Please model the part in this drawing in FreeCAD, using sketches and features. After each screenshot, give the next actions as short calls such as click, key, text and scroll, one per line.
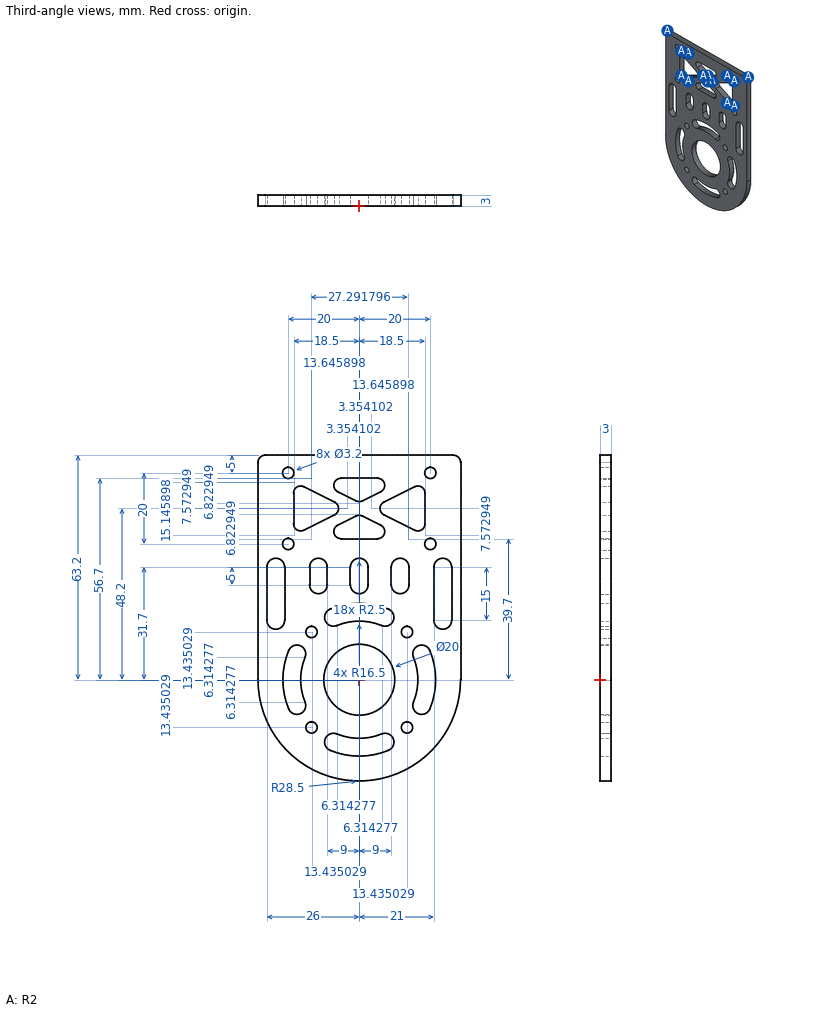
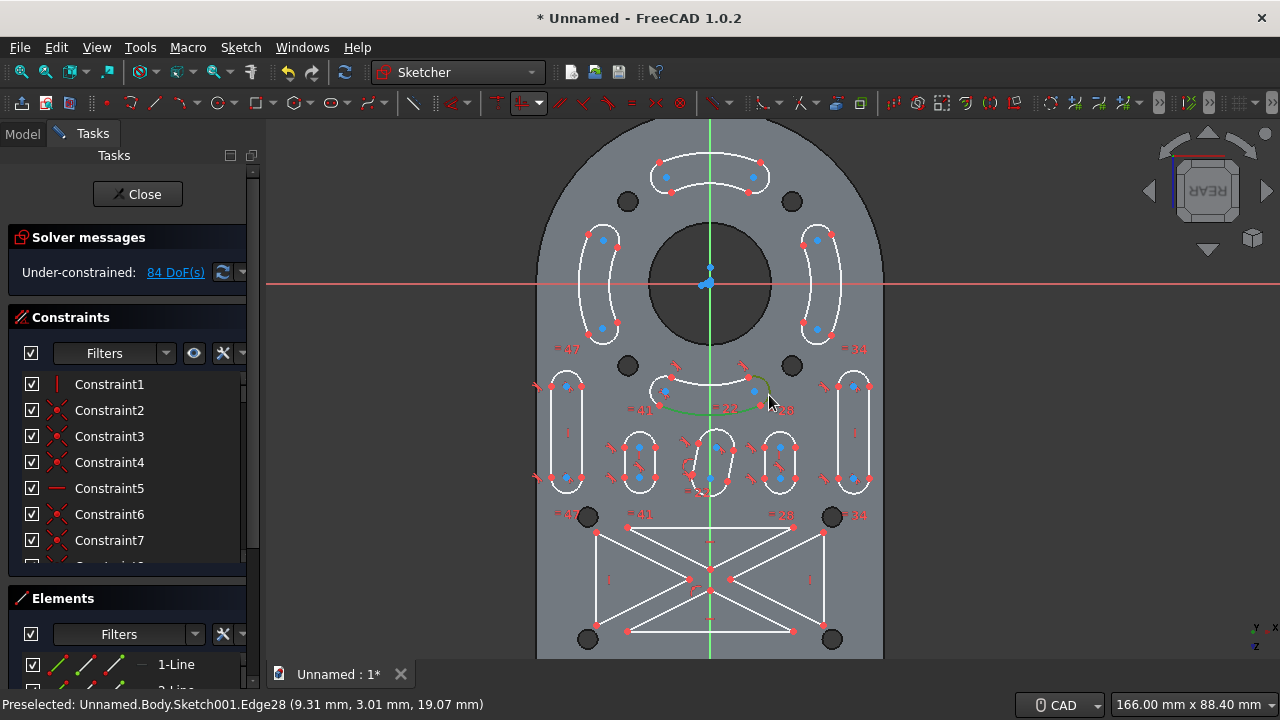
key(t)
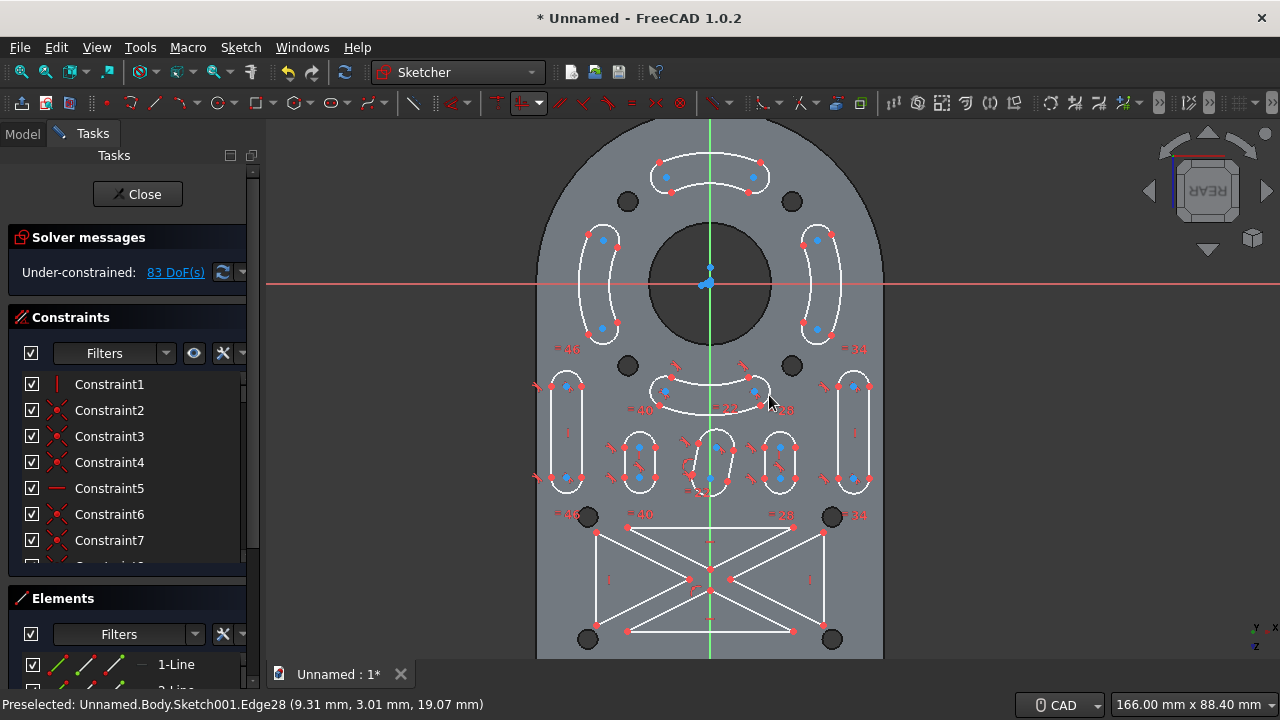
click(611, 269)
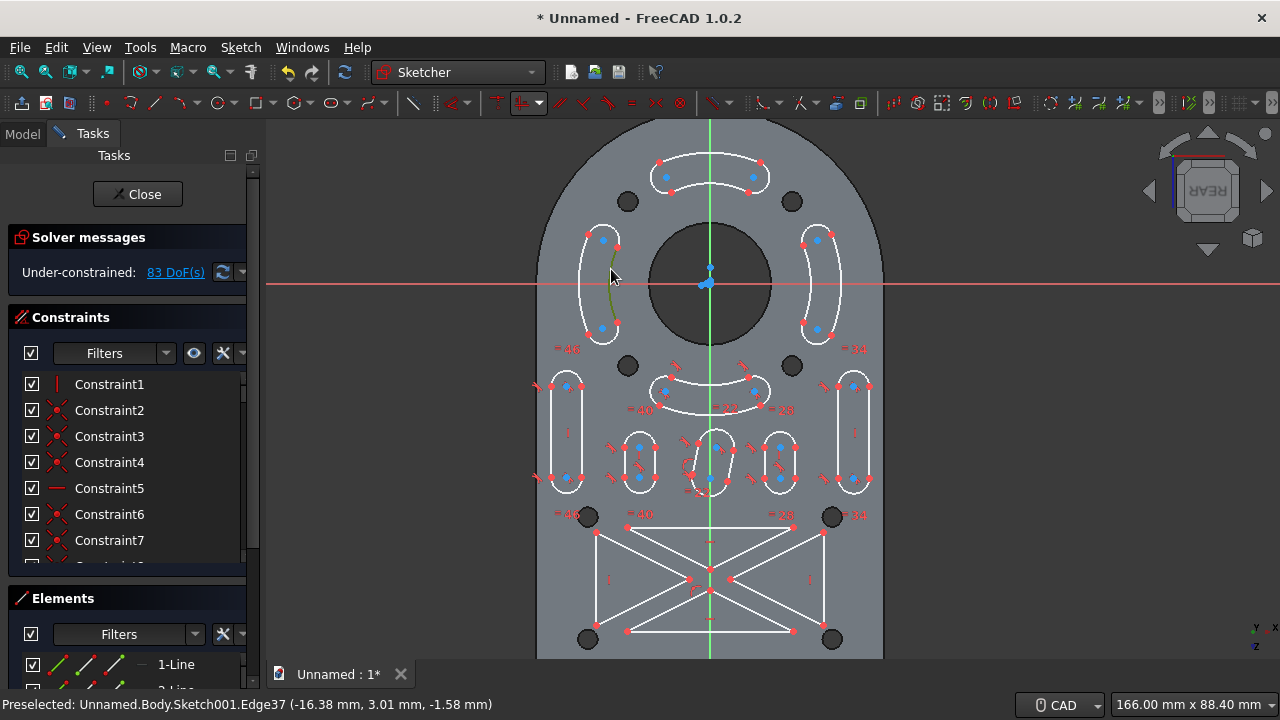
click(617, 233)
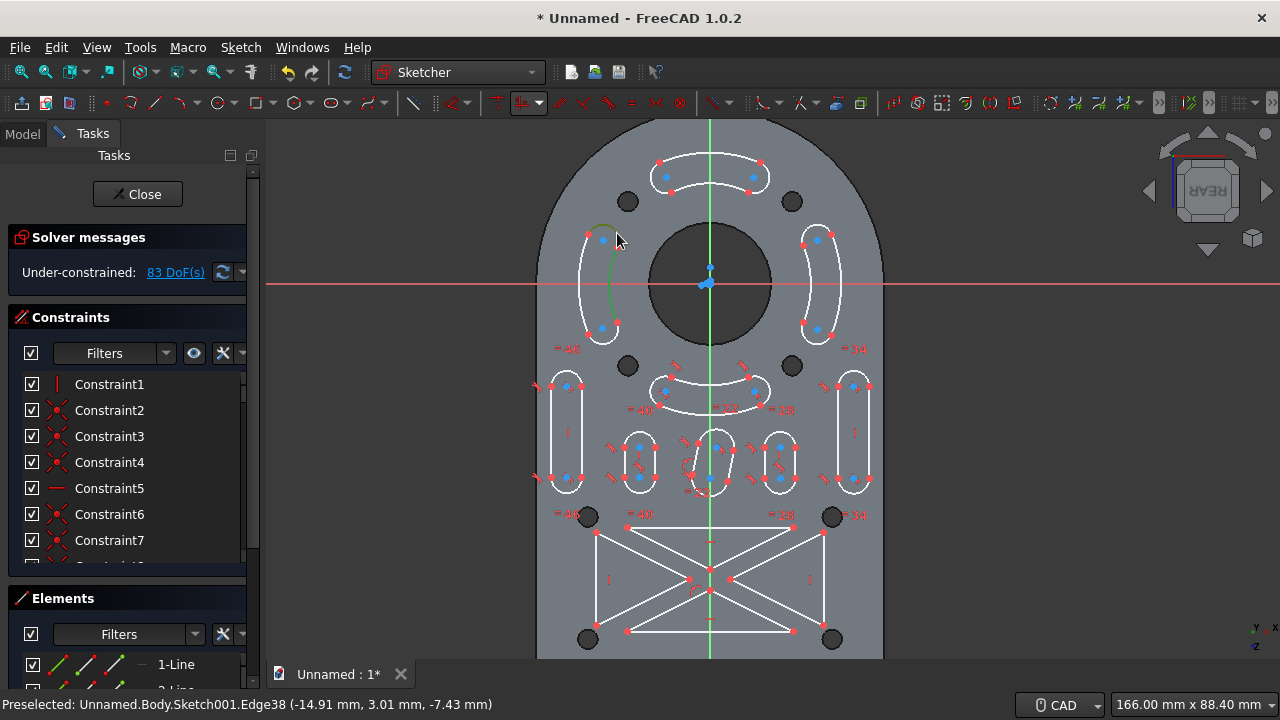
click(608, 104)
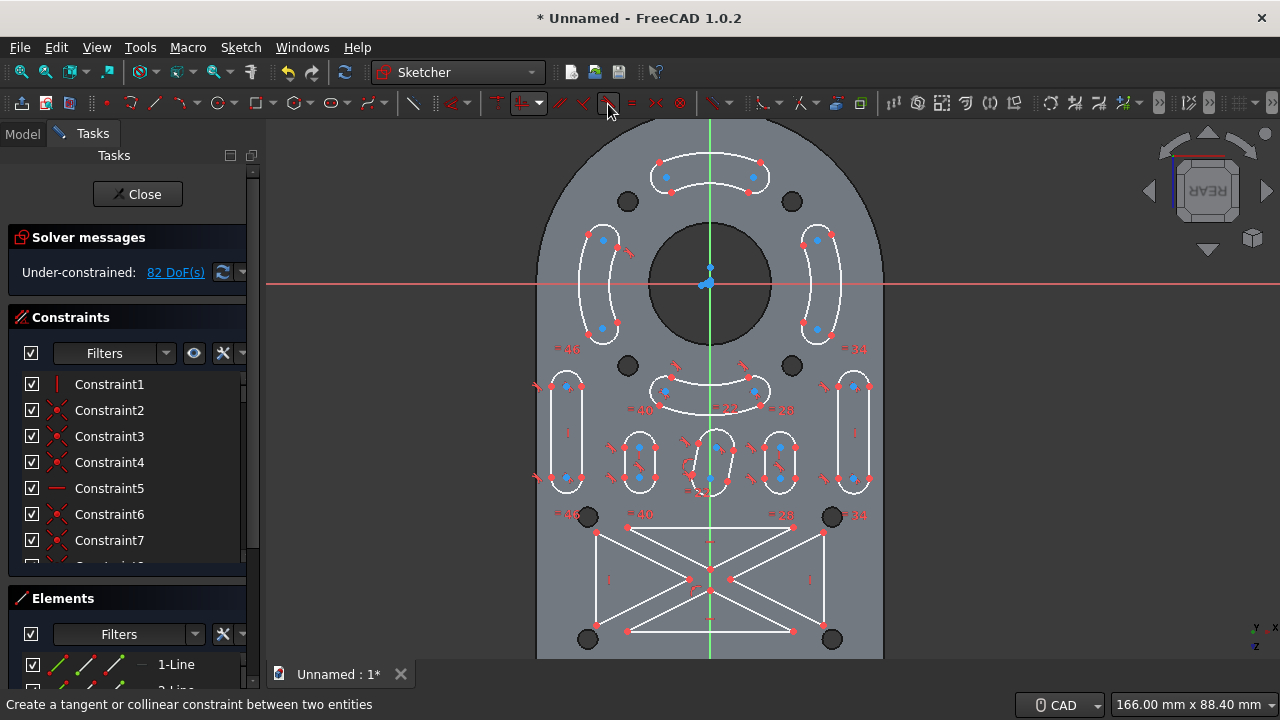
click(611, 269)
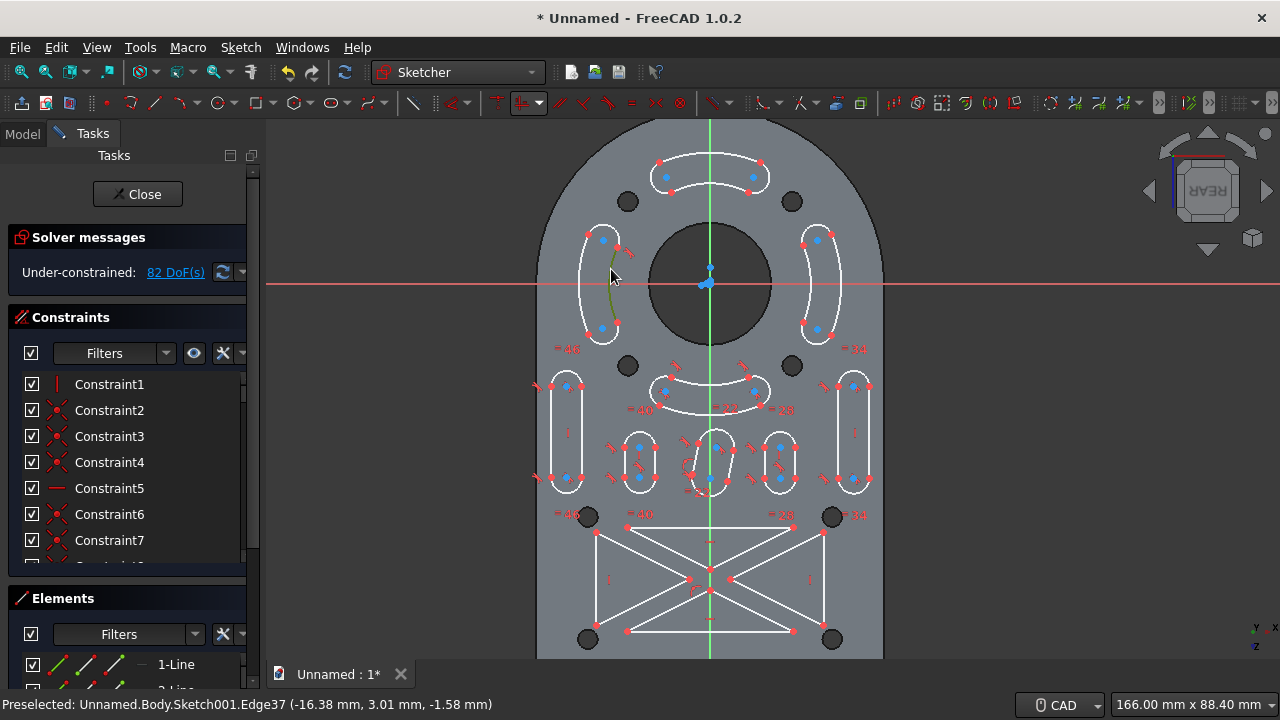
click(599, 344)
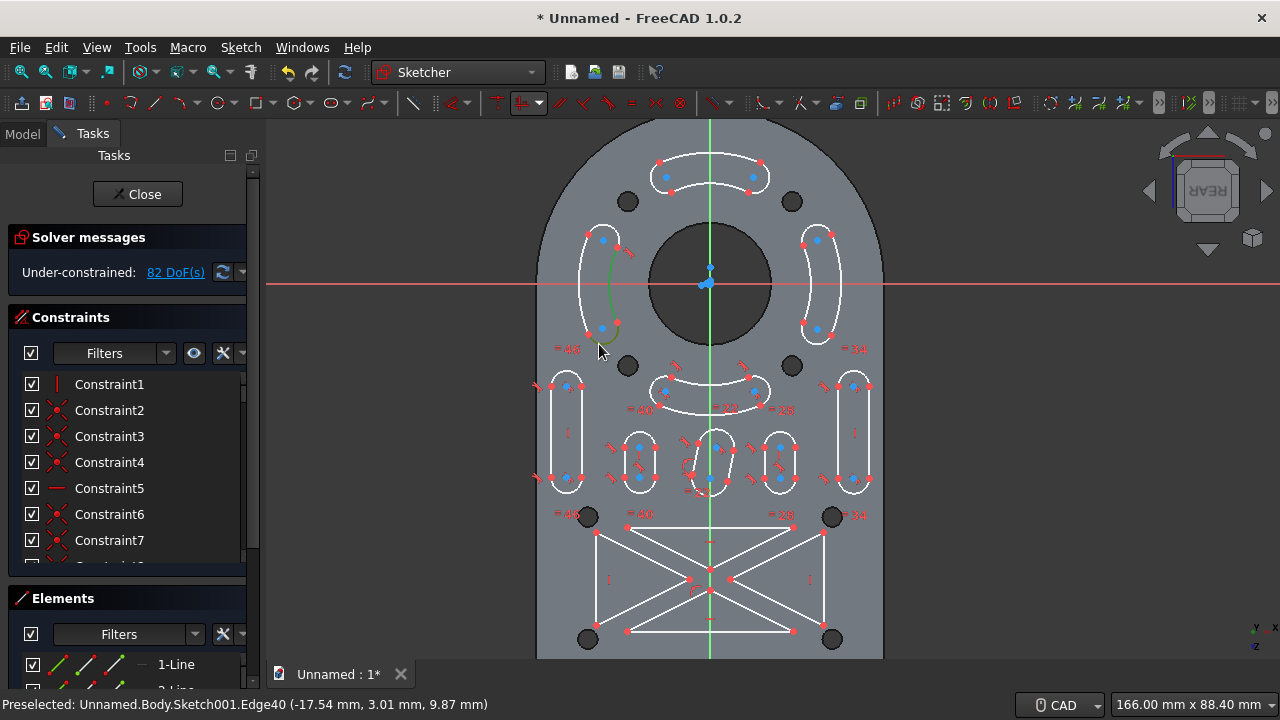
key(t)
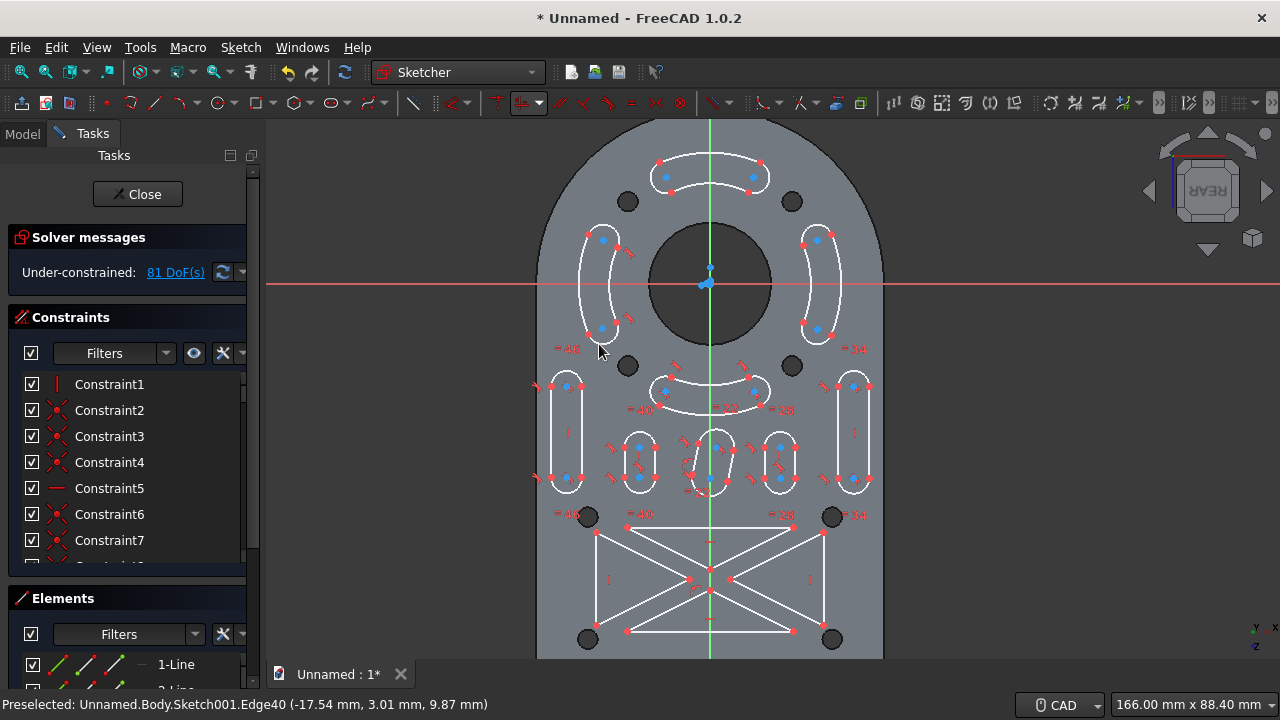
click(617, 233)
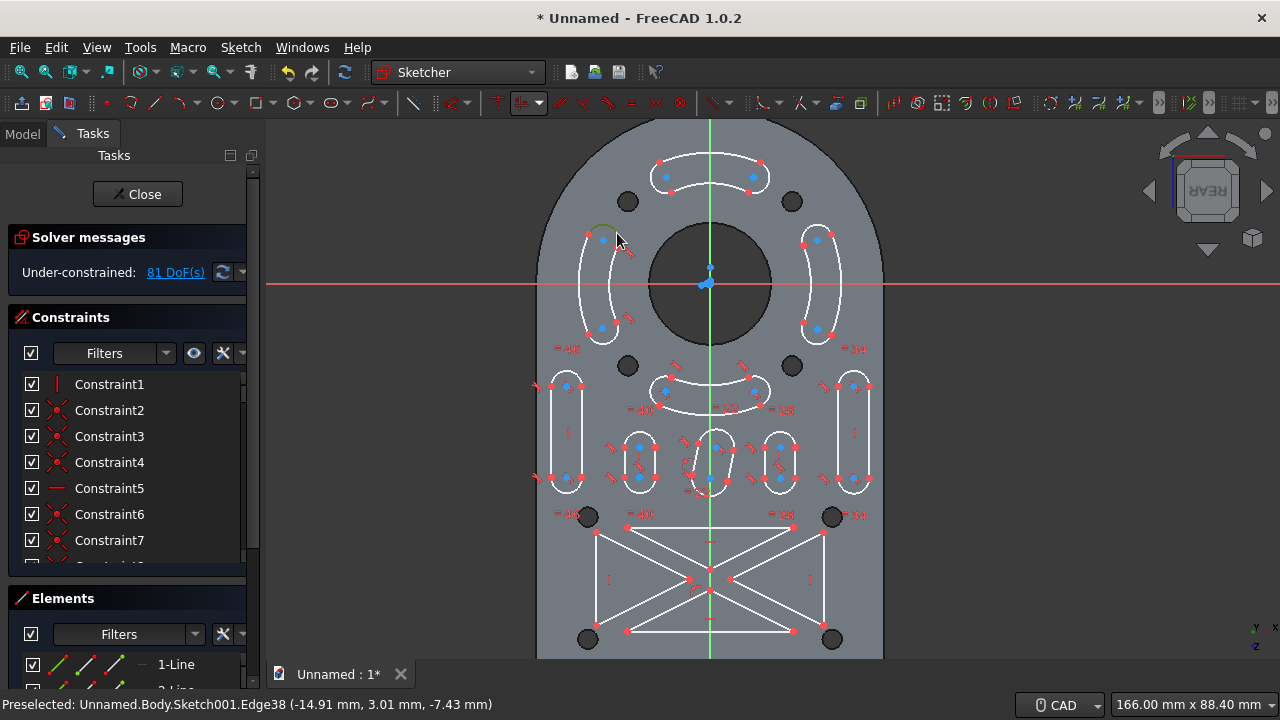
click(580, 264)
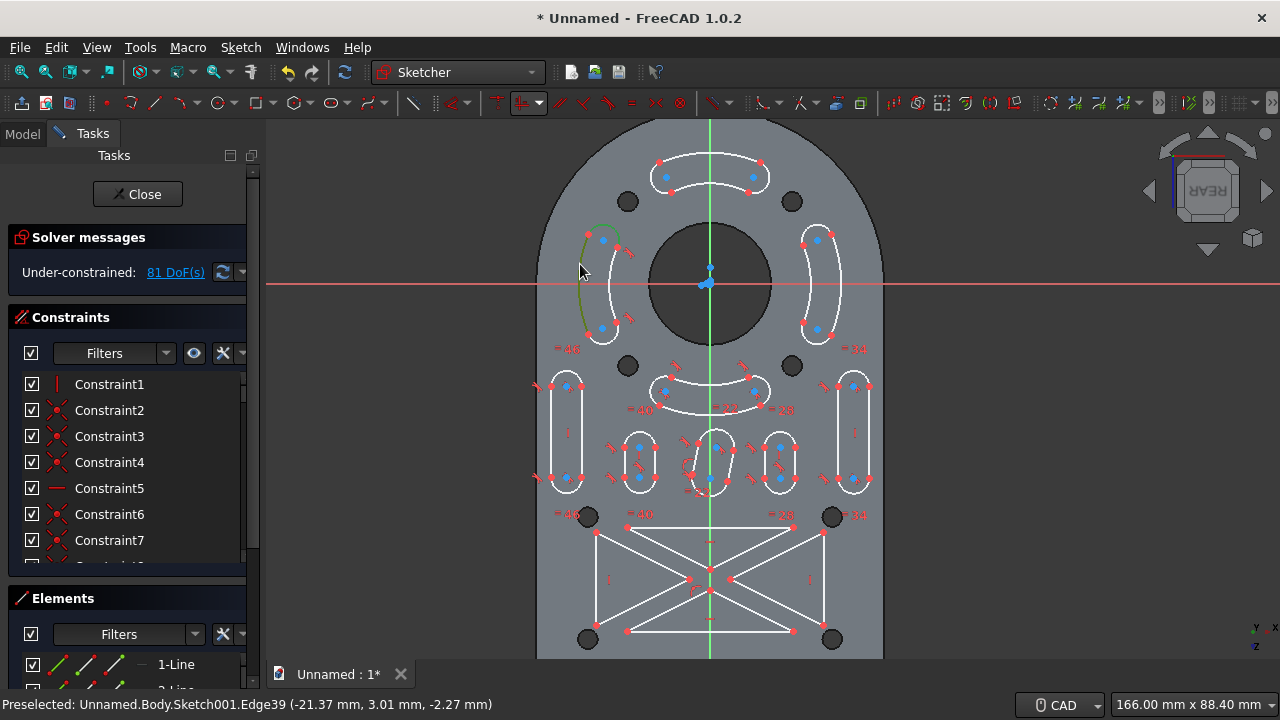
key(t)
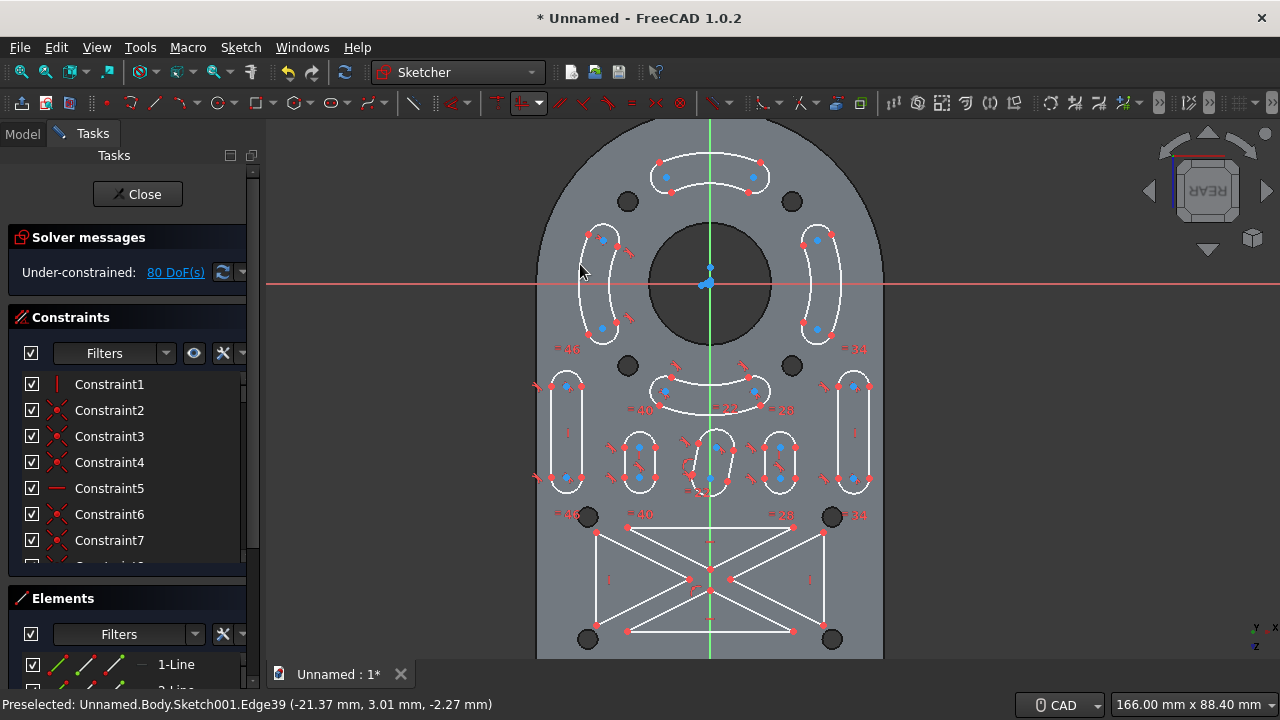
click(580, 264)